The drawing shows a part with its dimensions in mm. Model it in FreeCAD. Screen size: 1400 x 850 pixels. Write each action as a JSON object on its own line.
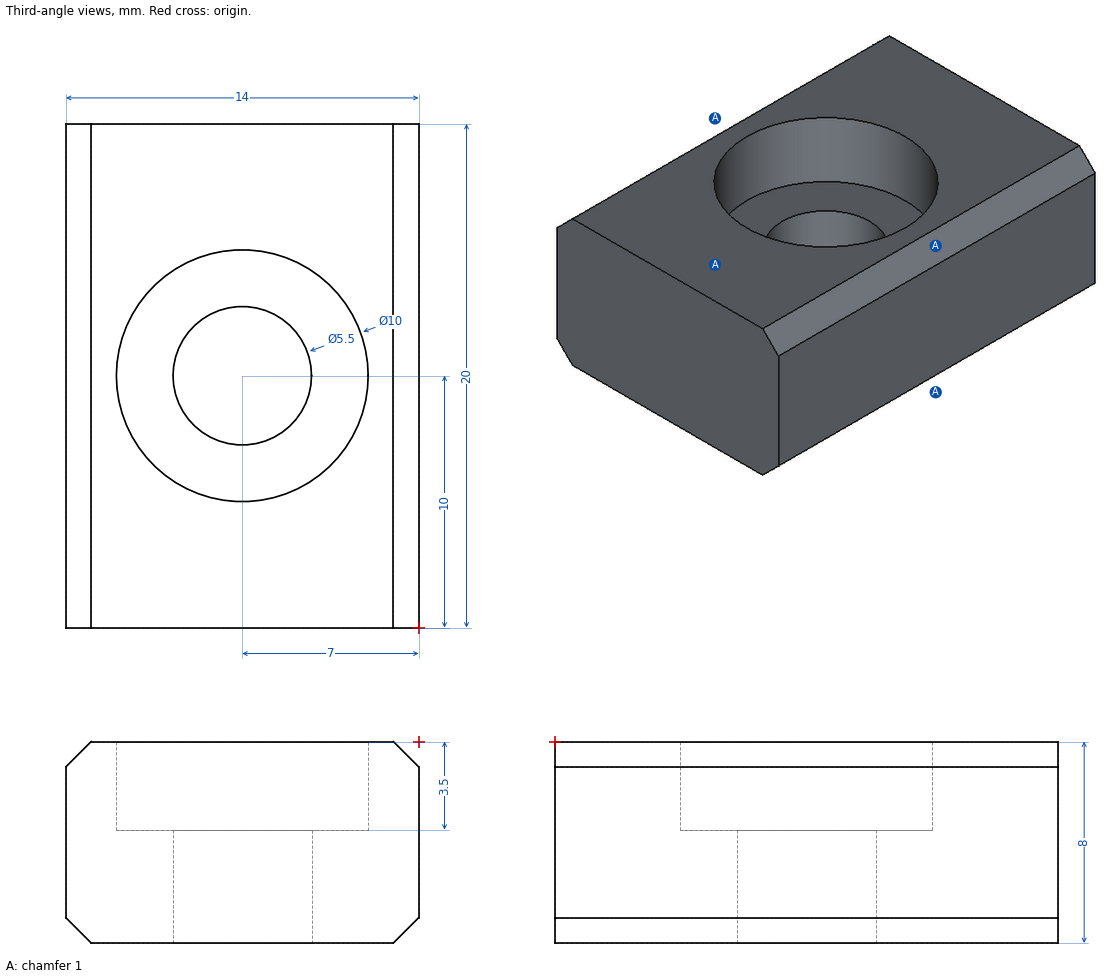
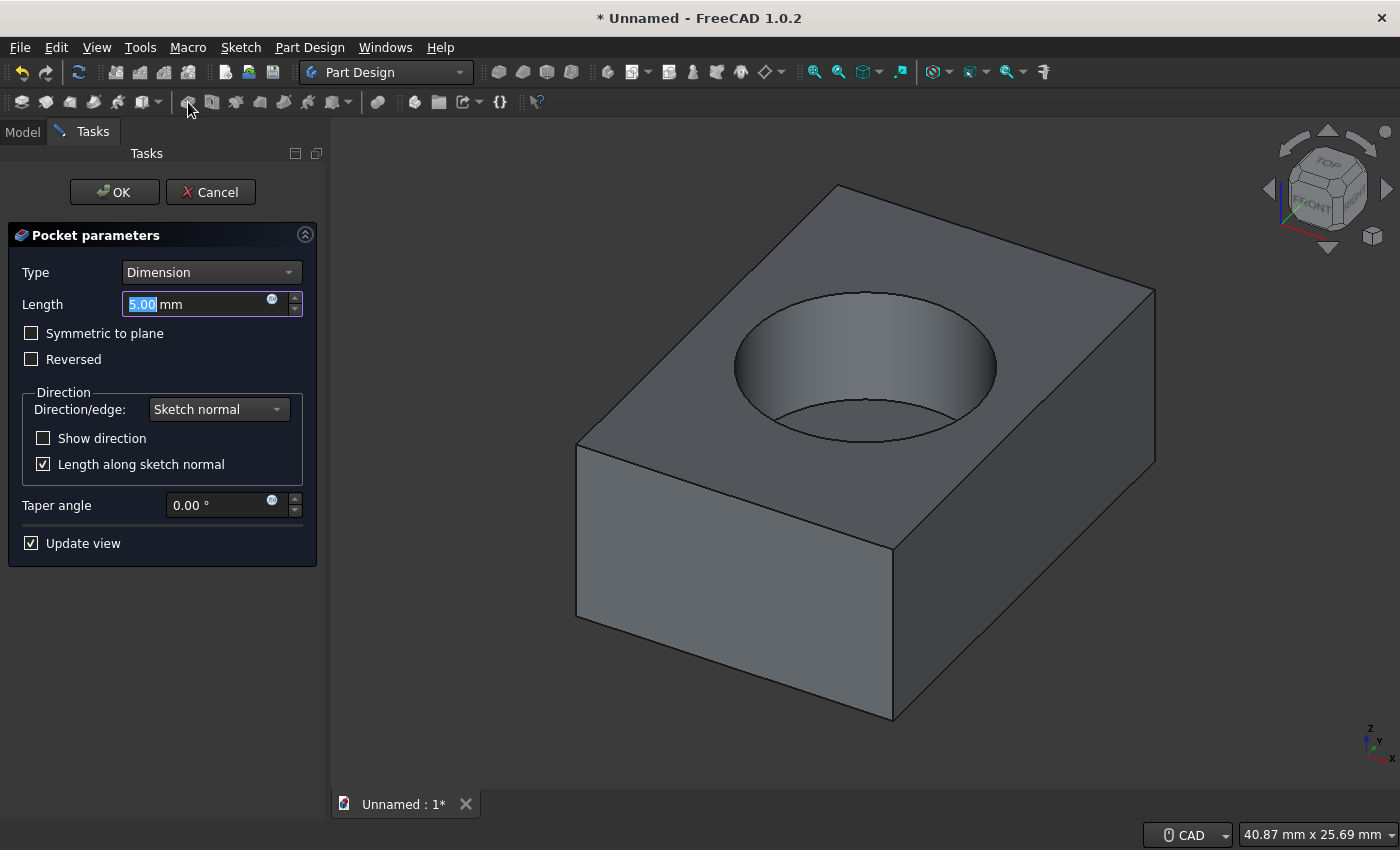
{"action": "type", "text": "3.5"}
{"action": "key", "text": "Tab"}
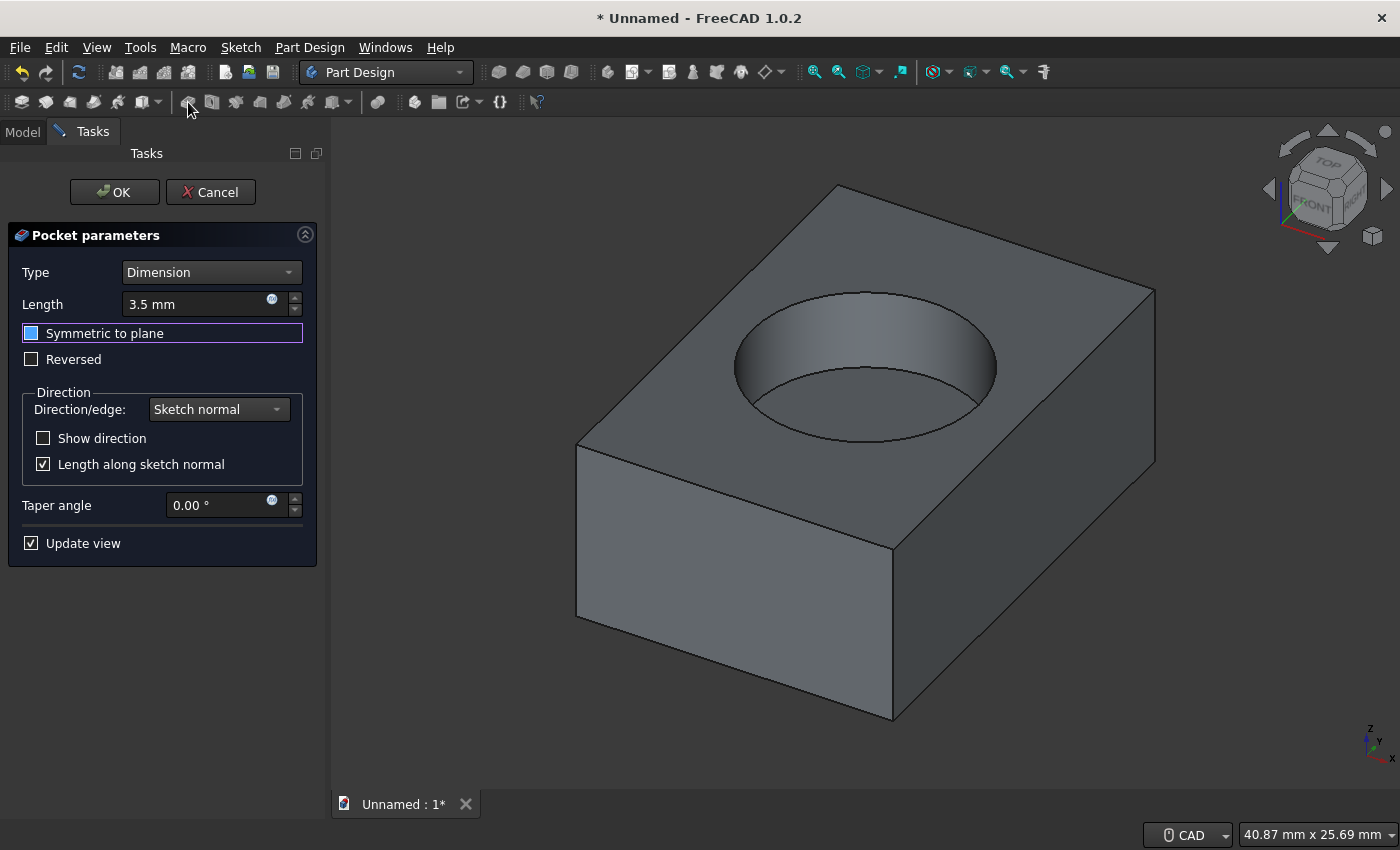
{"action": "left_click", "coordinate": [115, 192]}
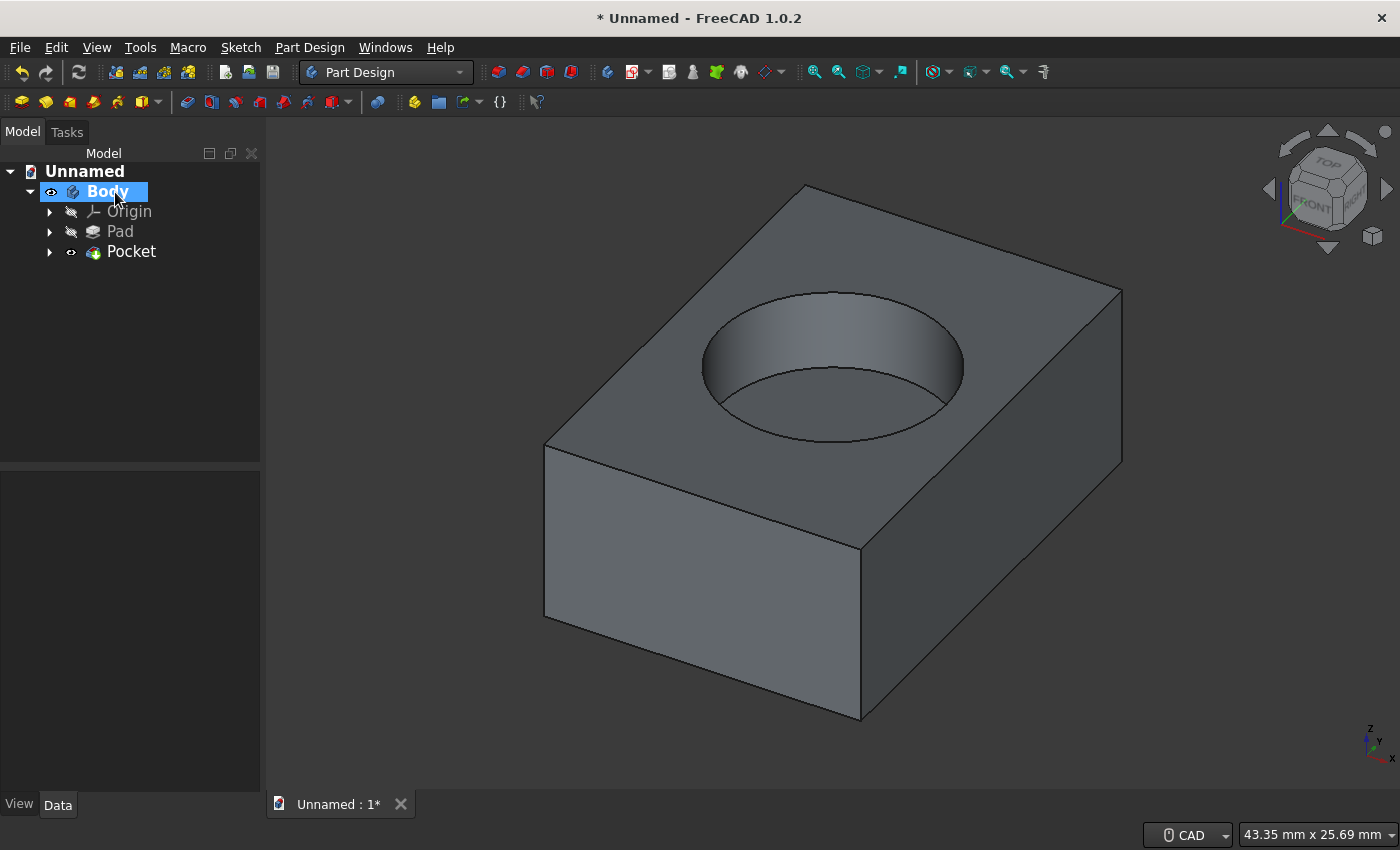
{"action": "left_click", "coordinate": [852, 423]}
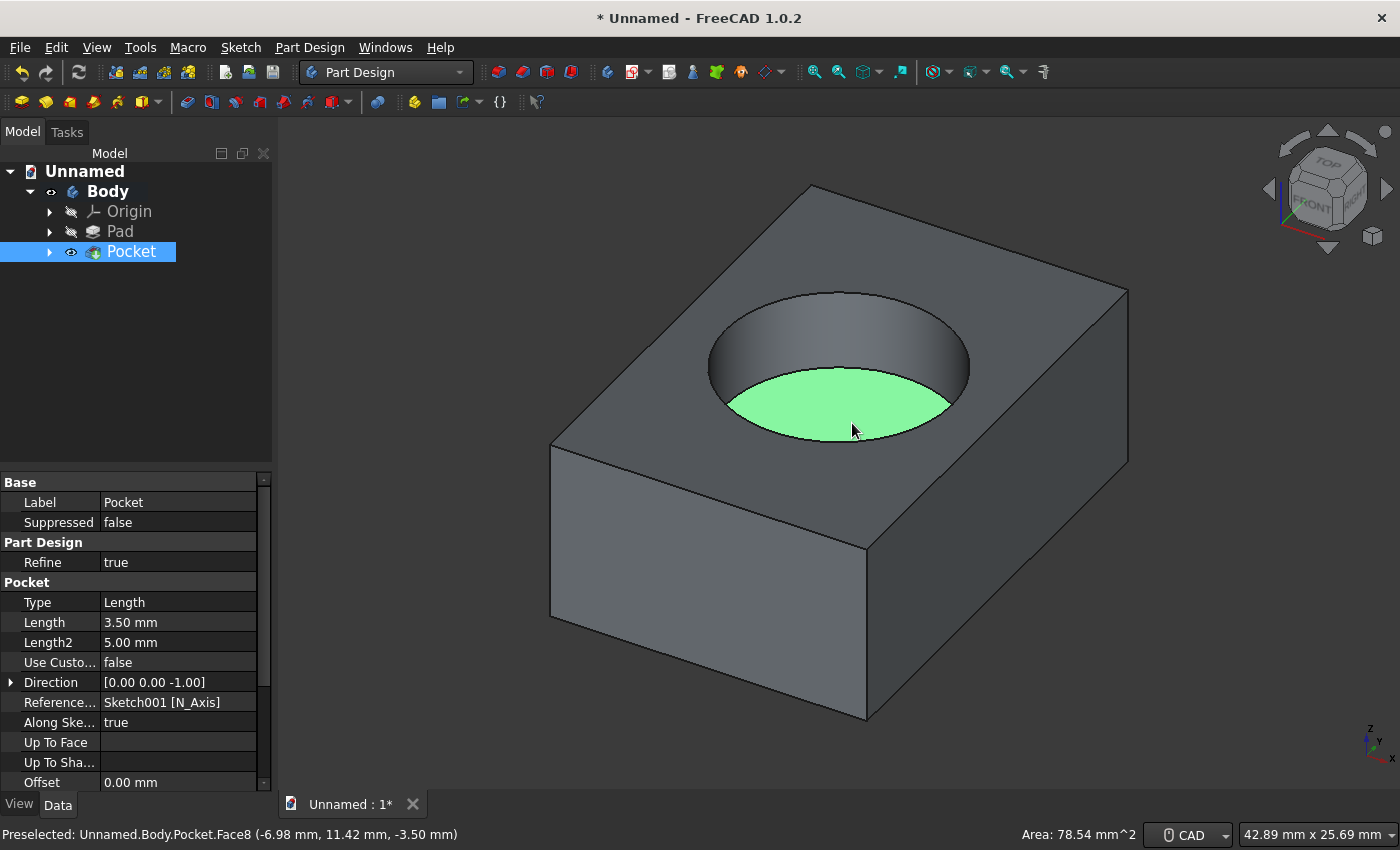
{"action": "left_click", "coordinate": [632, 72]}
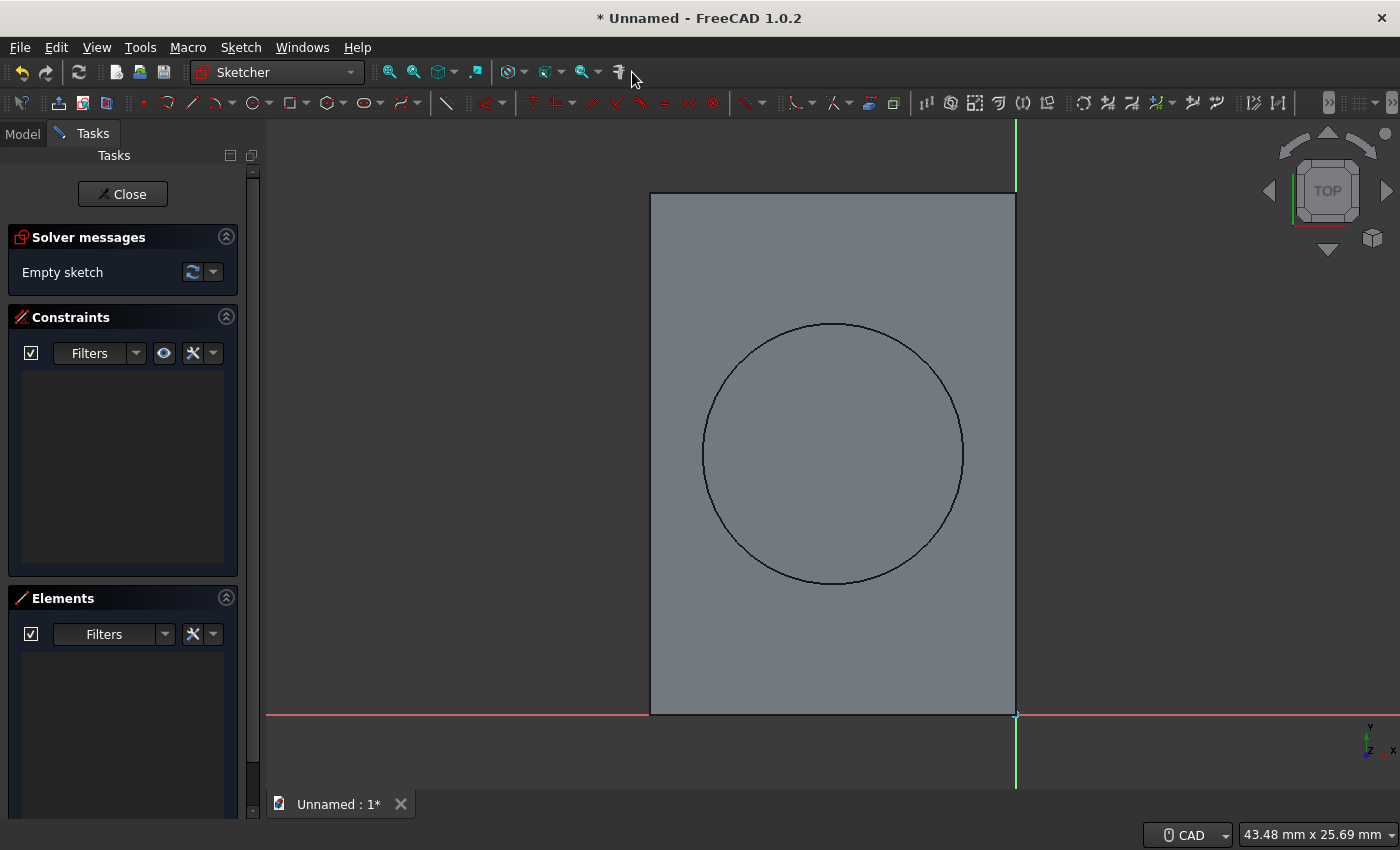
{"action": "key", "text": "q s"}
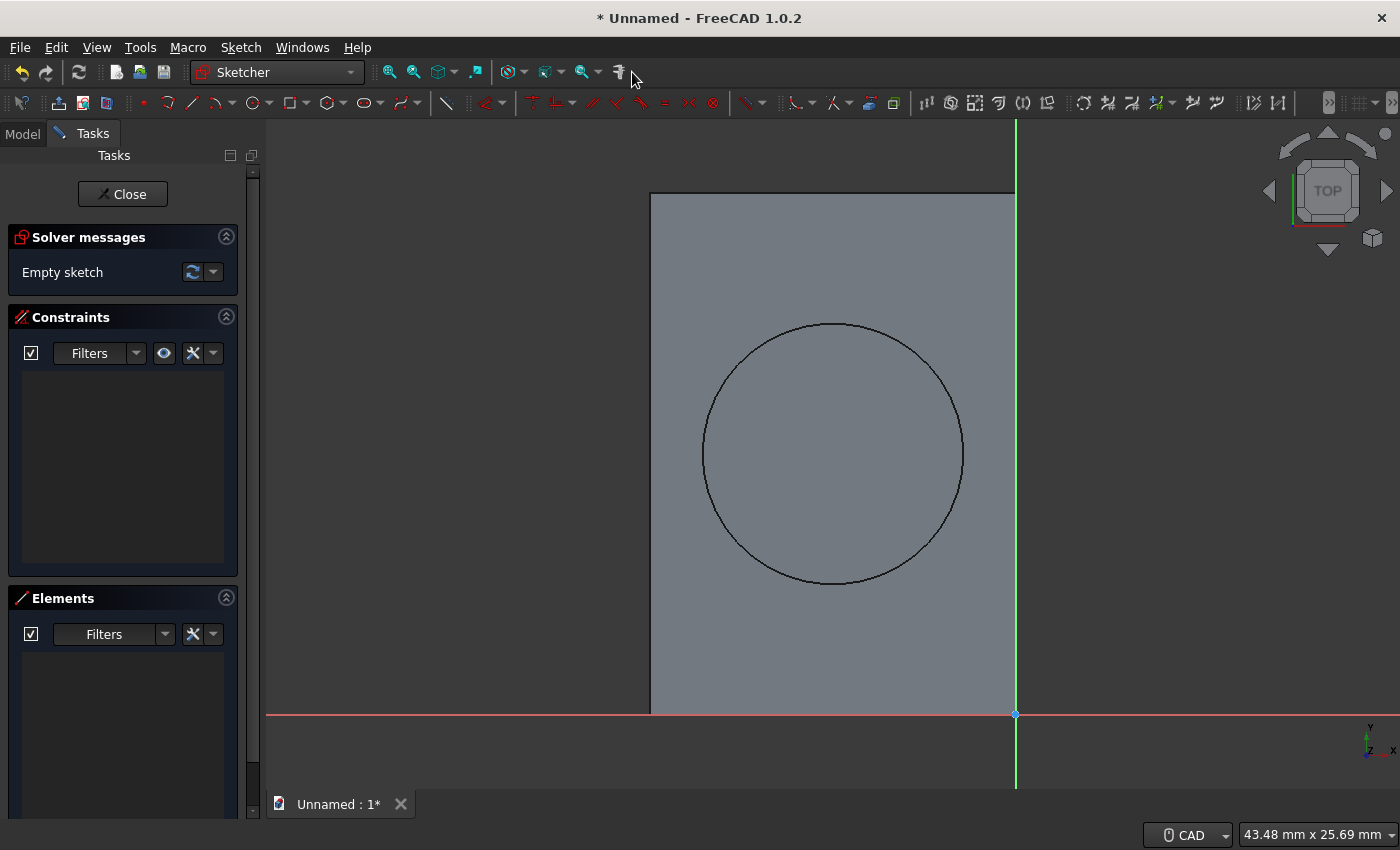
{"action": "left_click", "coordinate": [254, 104]}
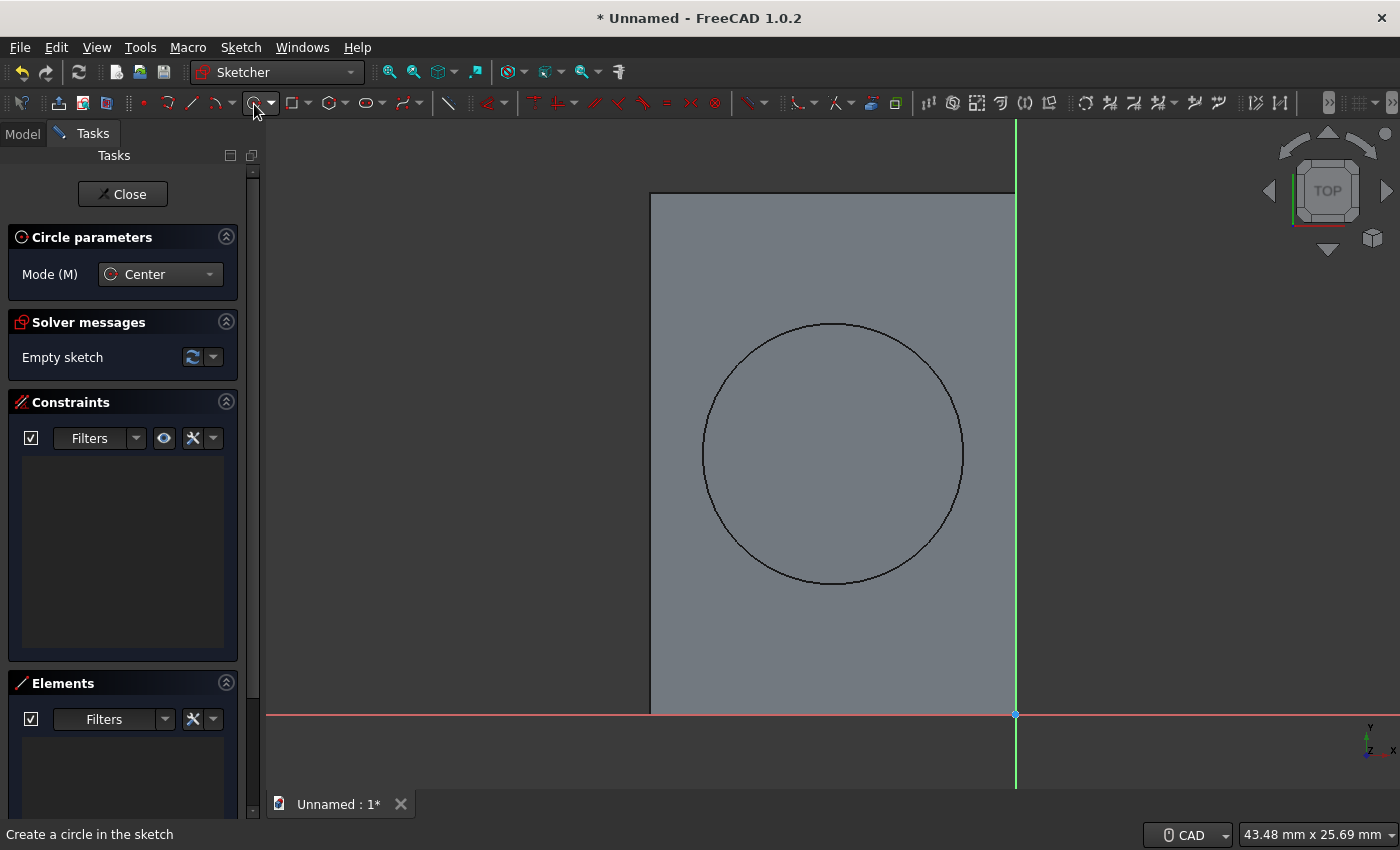
{"action": "left_click", "coordinate": [833, 454]}
{"action": "left_click", "coordinate": [884, 403]}
{"action": "key", "text": "Escape"}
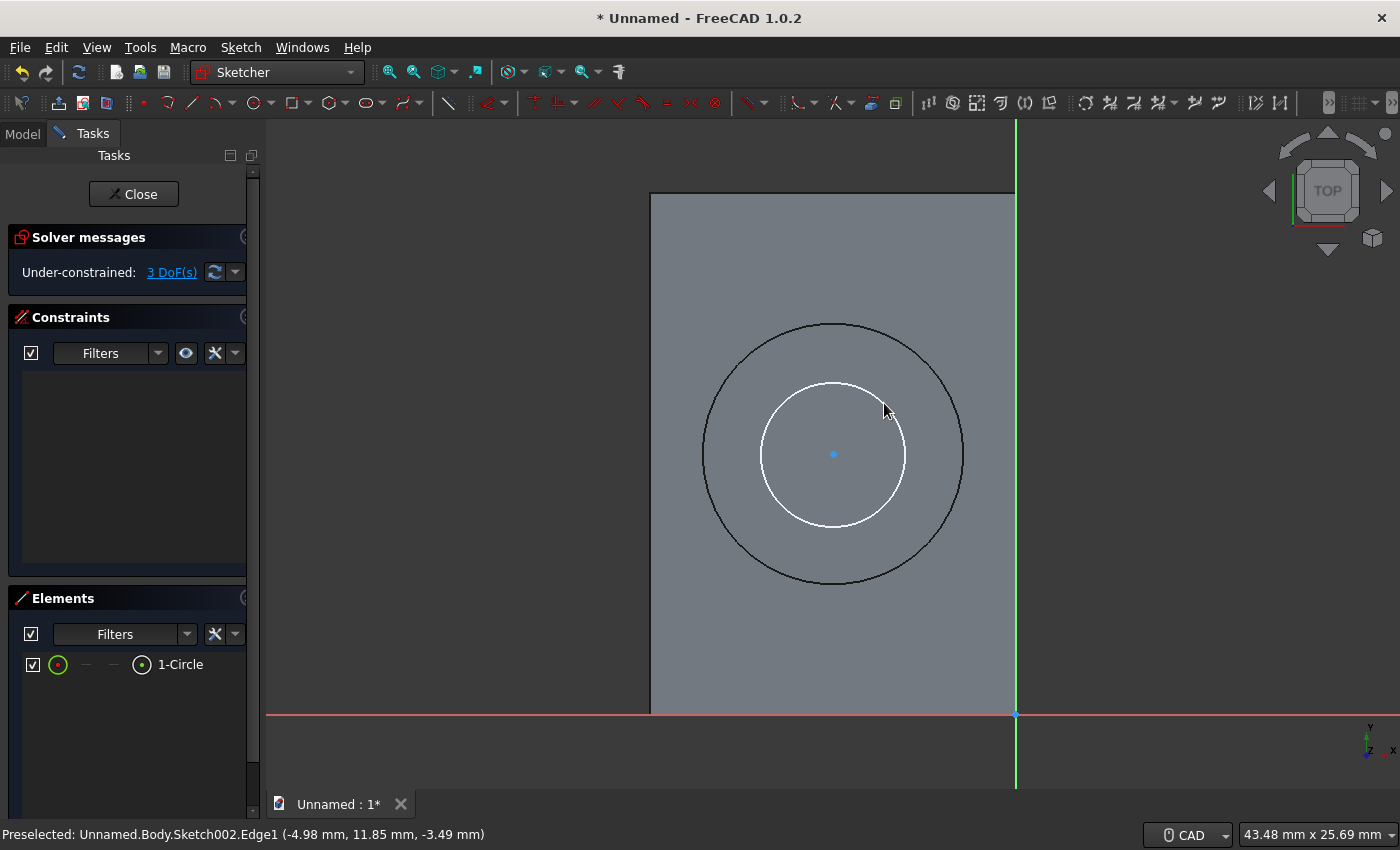
{"action": "key", "text": "d"}